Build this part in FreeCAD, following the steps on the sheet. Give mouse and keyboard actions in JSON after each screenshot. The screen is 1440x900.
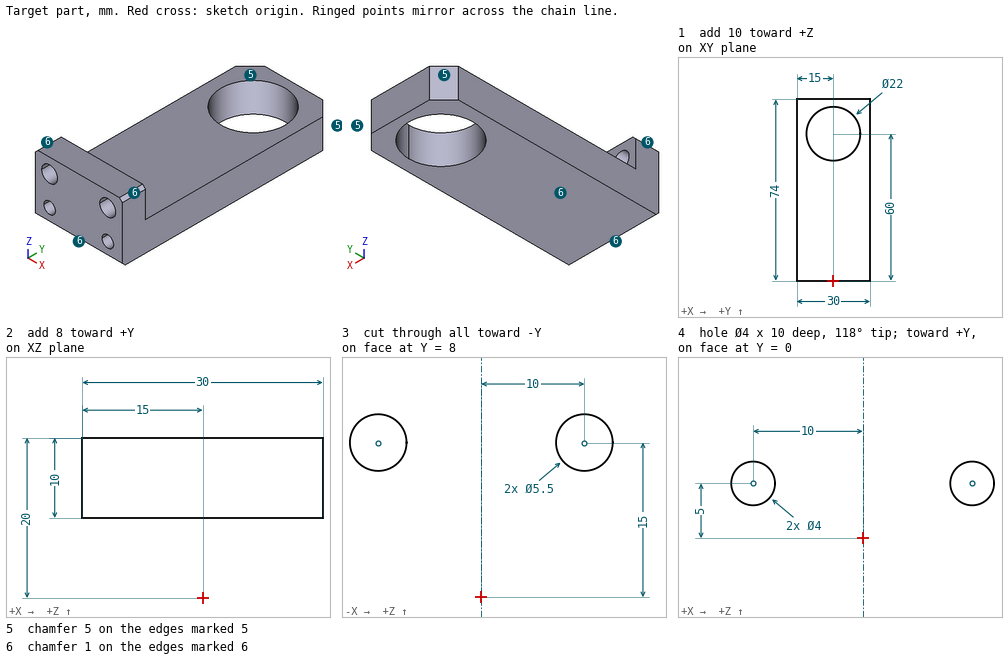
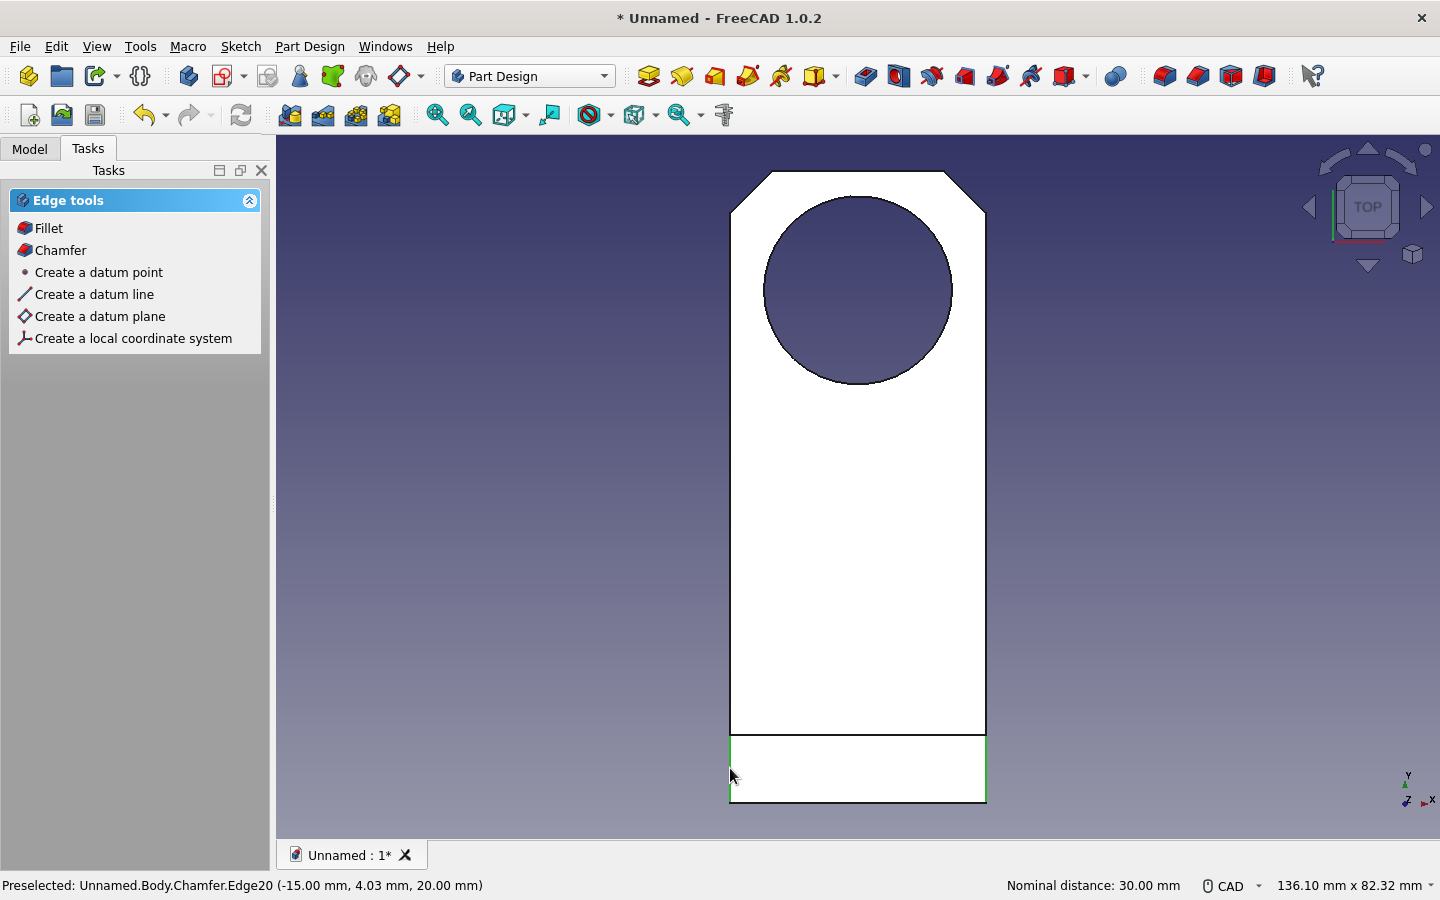
{"action": "key", "text": "1"}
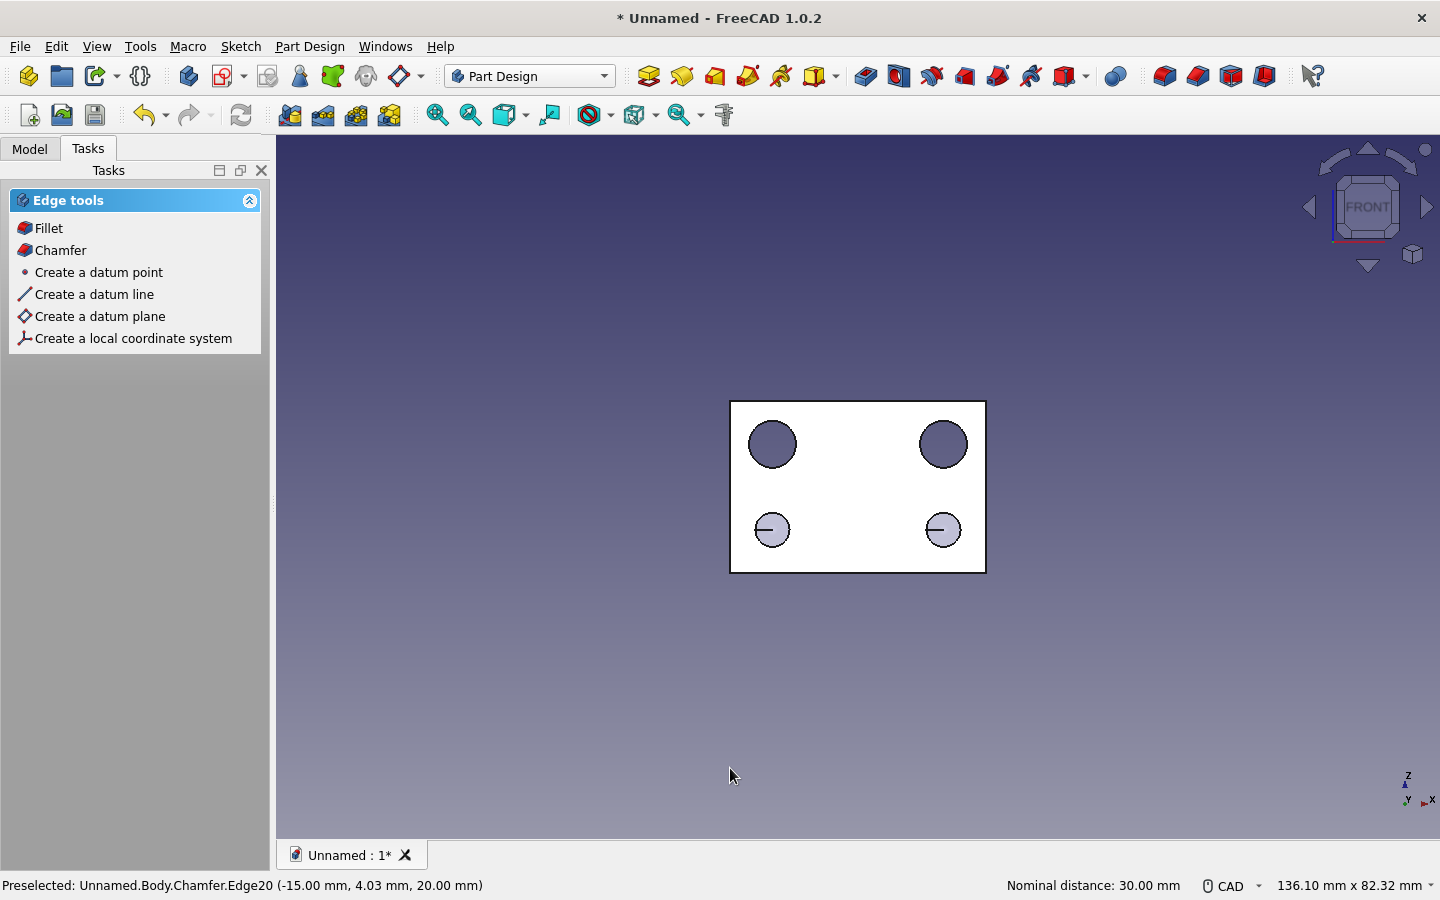
{"action": "left_click", "coordinate": [438, 116]}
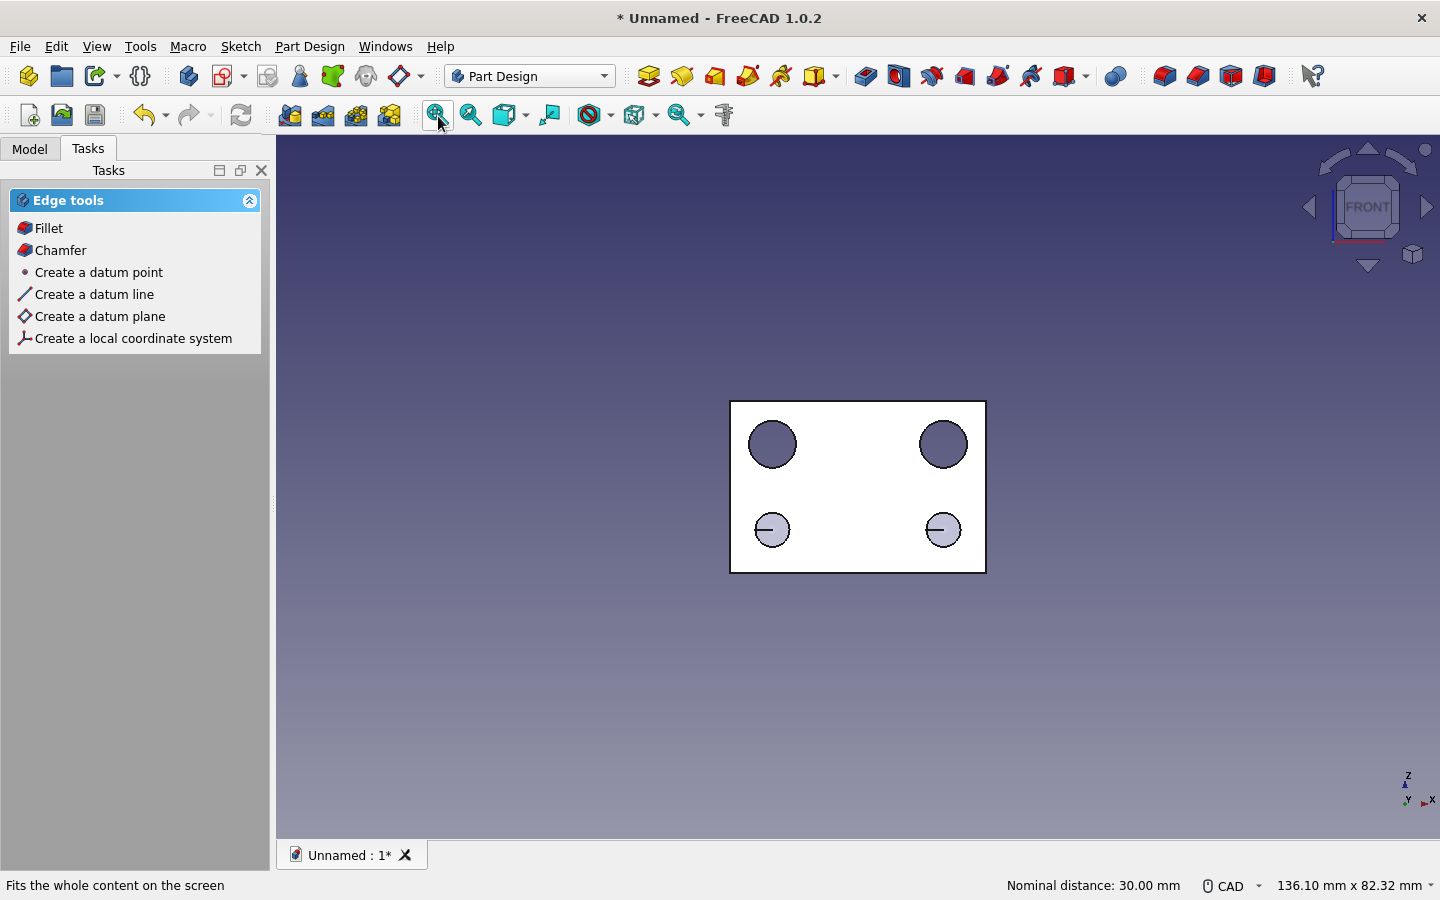
{"action": "left_click", "coordinate": [858, 572], "text": "ctrl"}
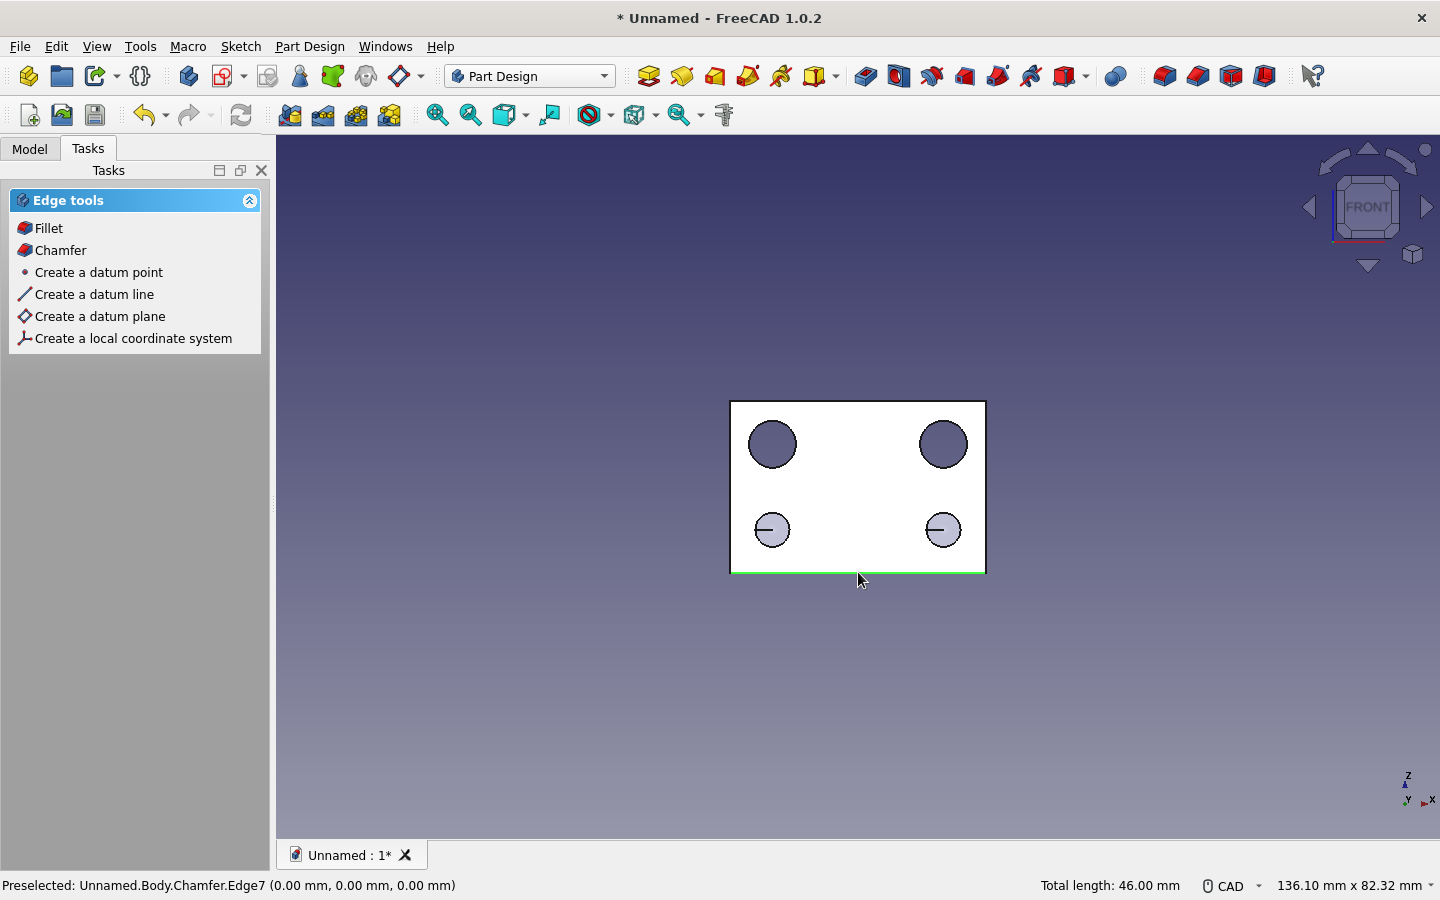
{"action": "left_click", "coordinate": [1198, 76]}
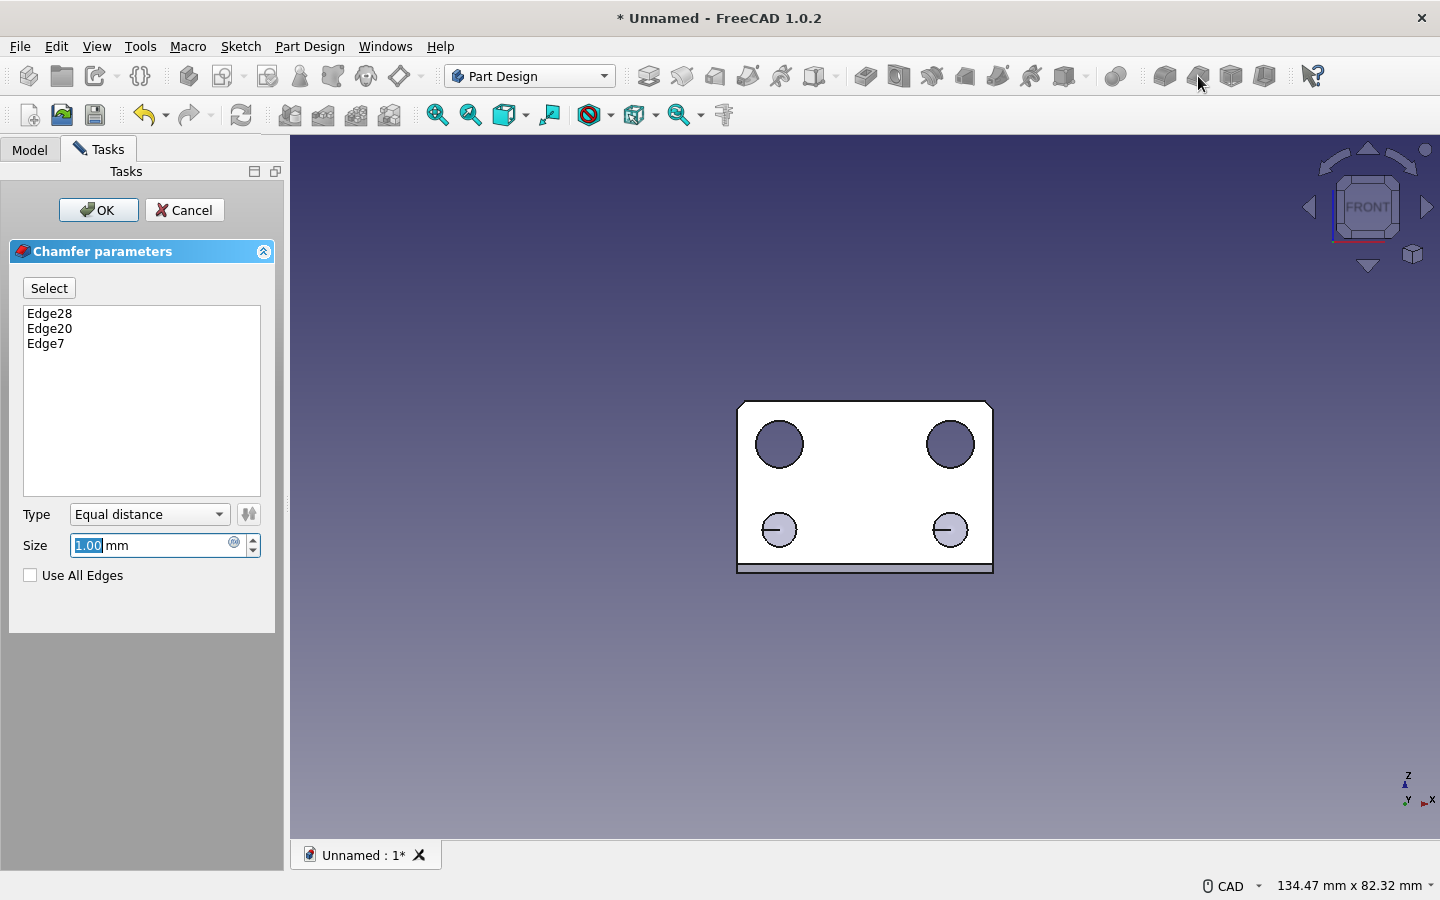
{"action": "type", "text": "1"}
{"action": "key", "text": "Tab"}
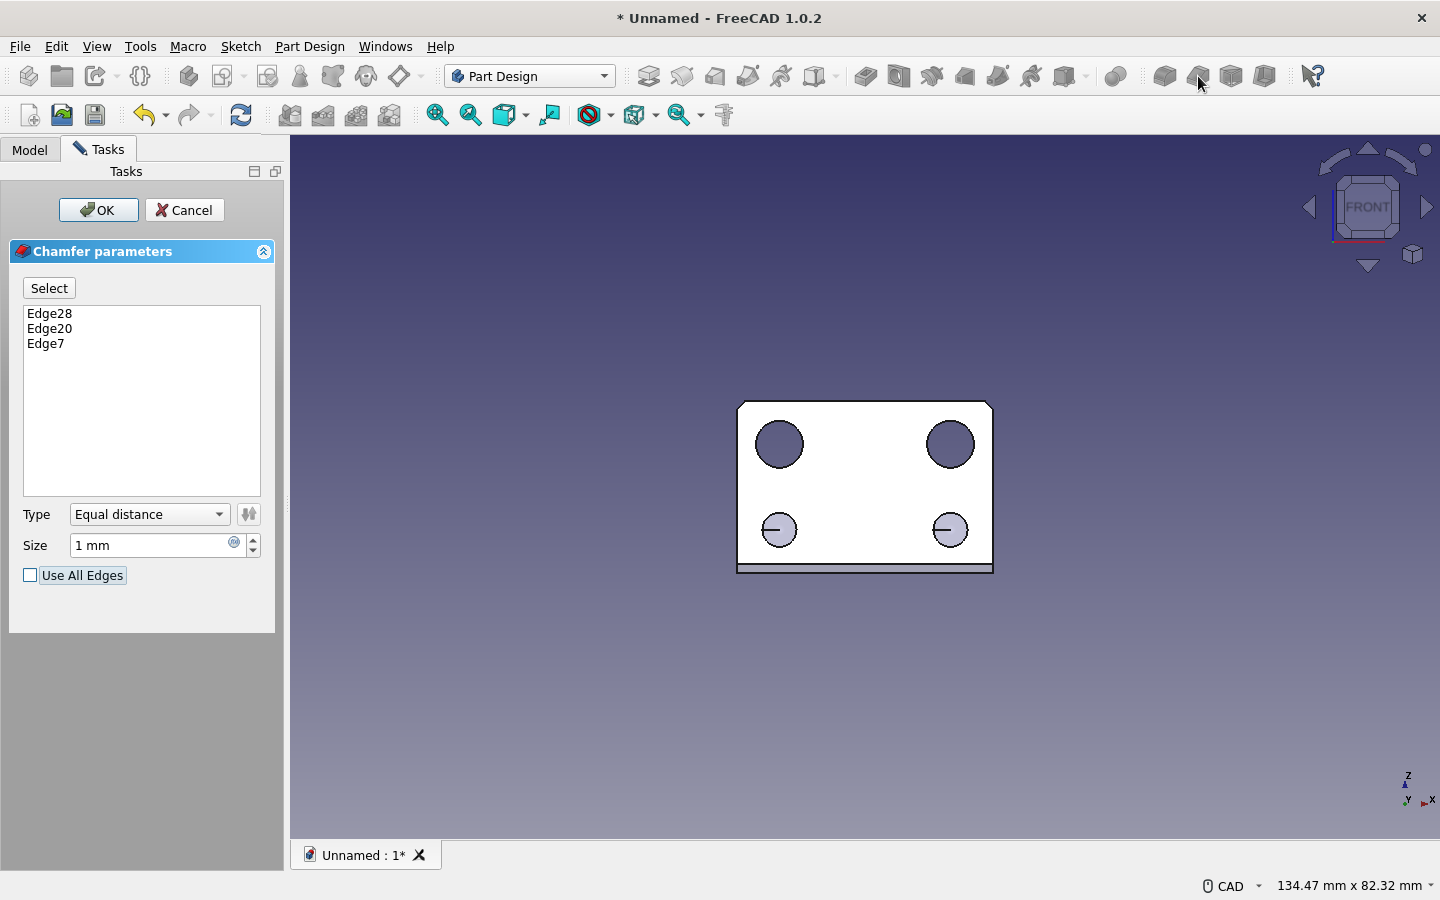
{"action": "left_click", "coordinate": [99, 210]}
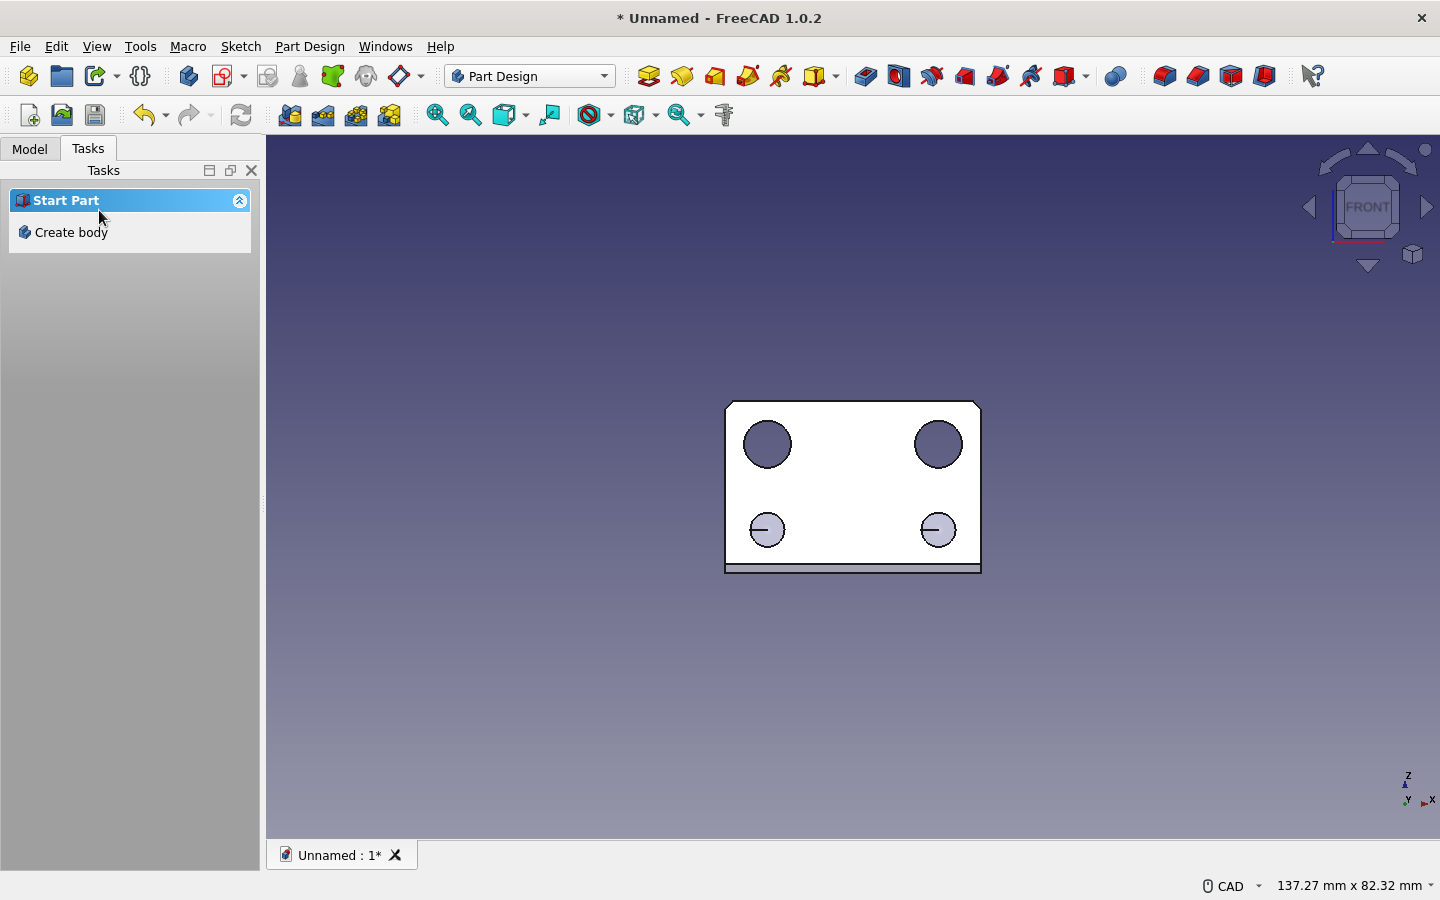
{"action": "key", "text": "0"}